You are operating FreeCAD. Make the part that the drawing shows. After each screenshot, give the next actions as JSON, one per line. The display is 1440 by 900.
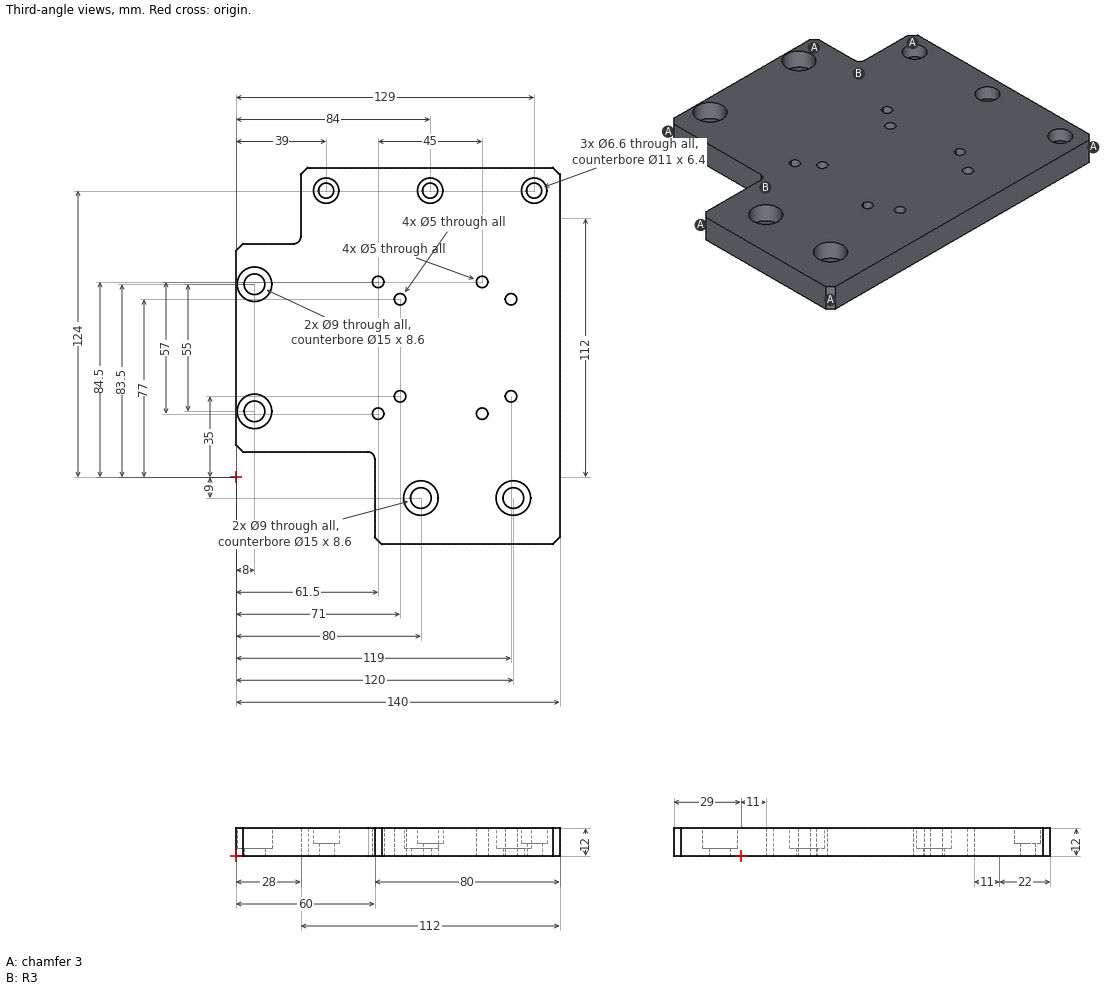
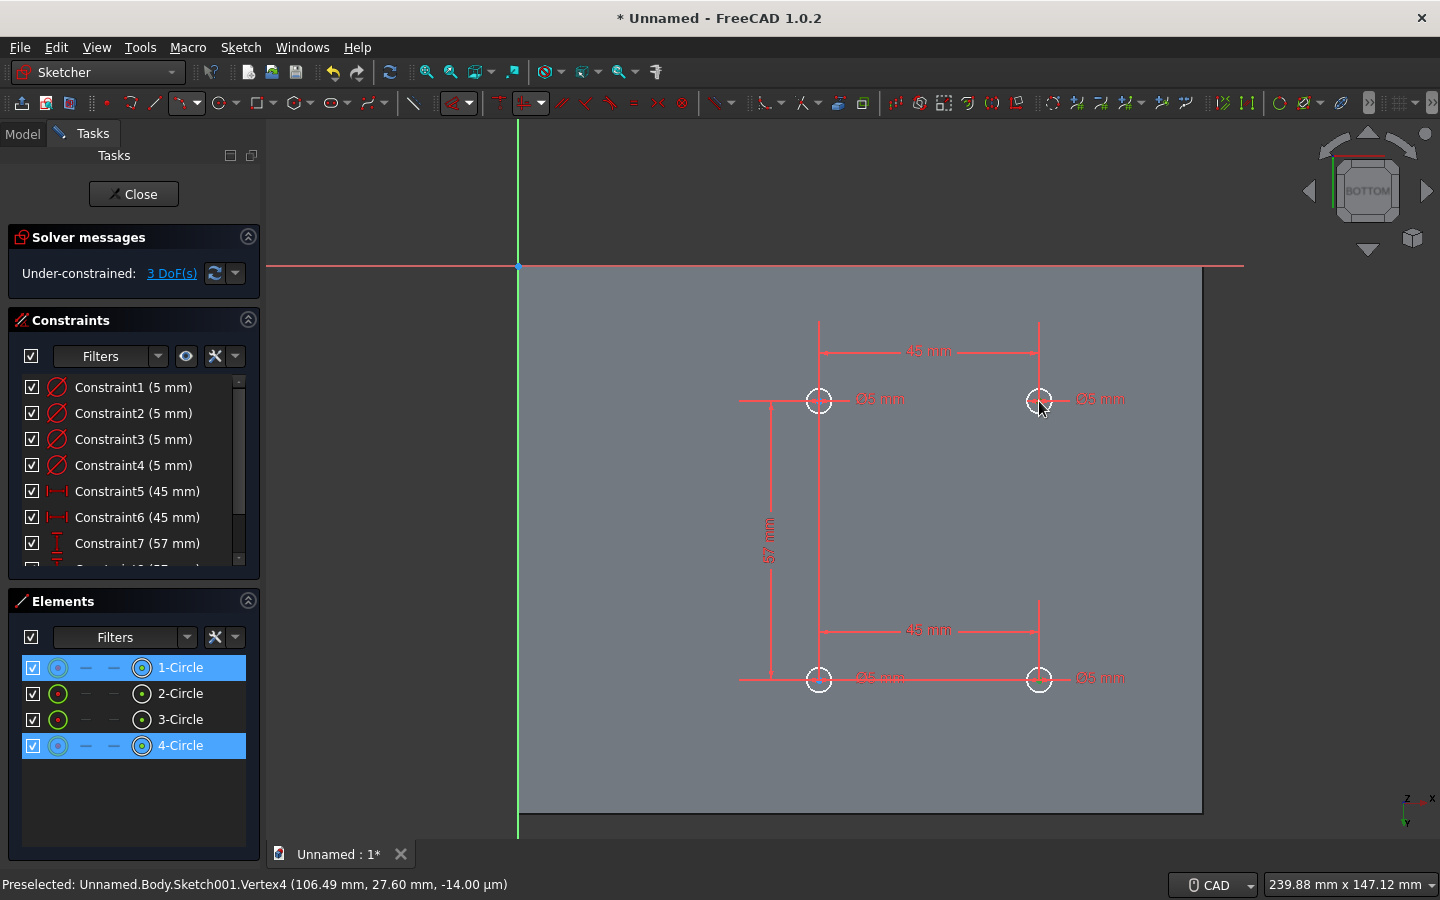
{"action": "left_click", "coordinate": [472, 104]}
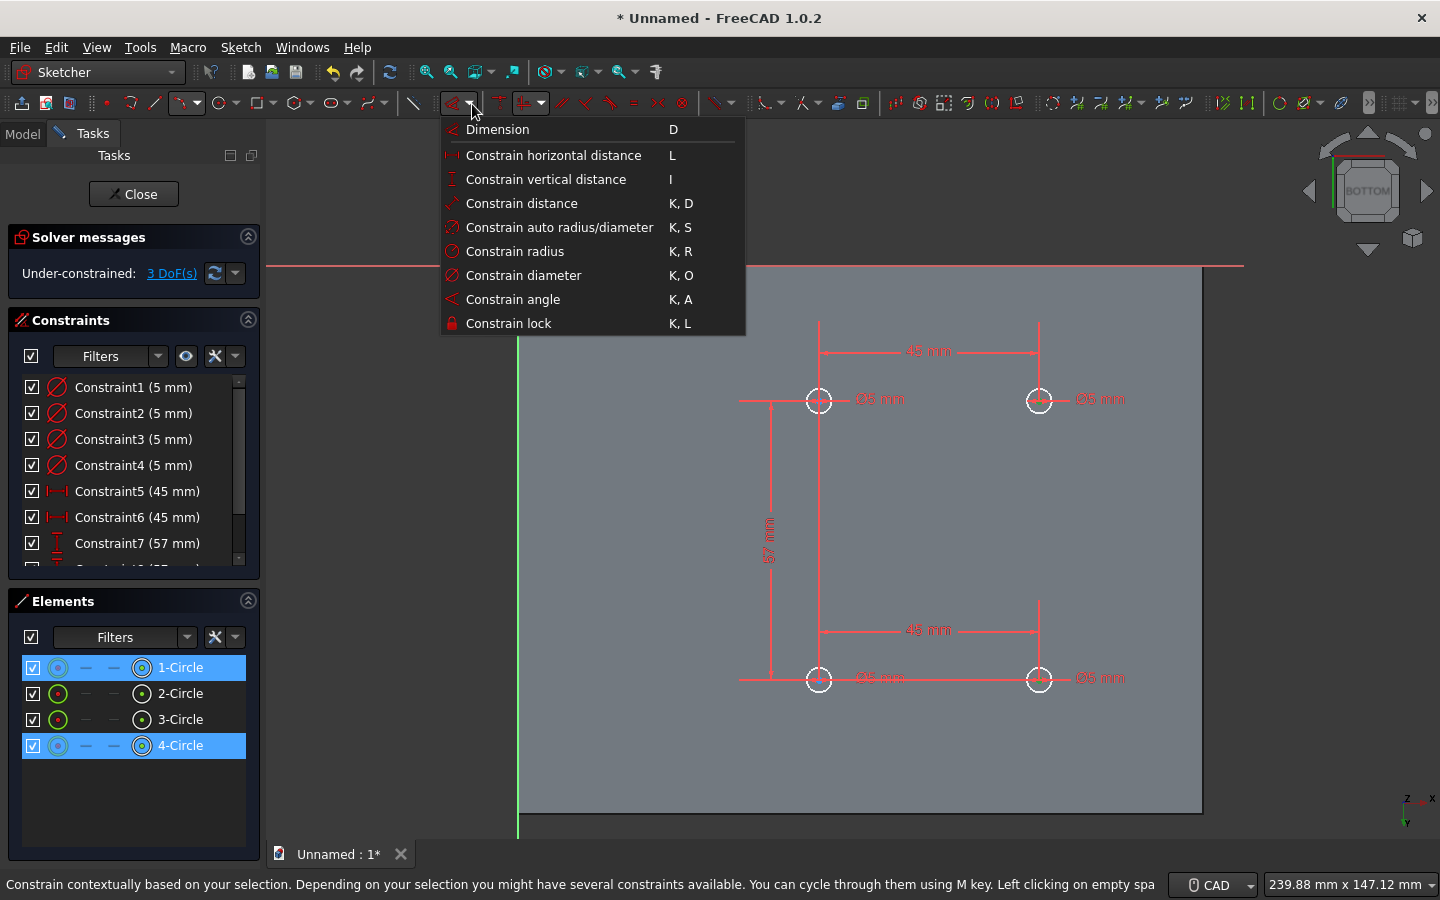
{"action": "left_click", "coordinate": [593, 179]}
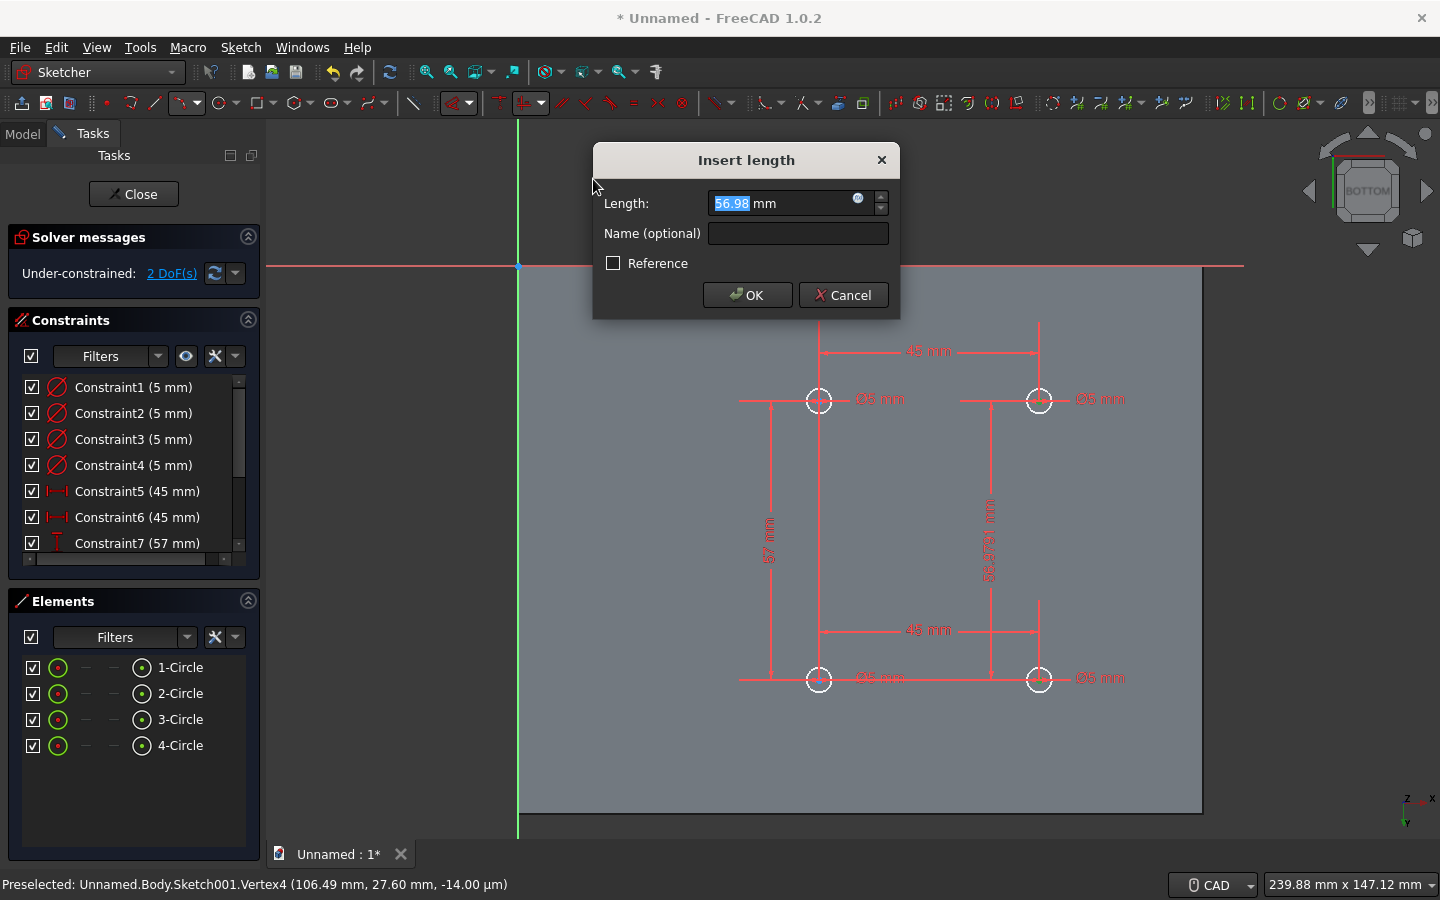
{"action": "type", "text": "57"}
{"action": "key", "text": "Return"}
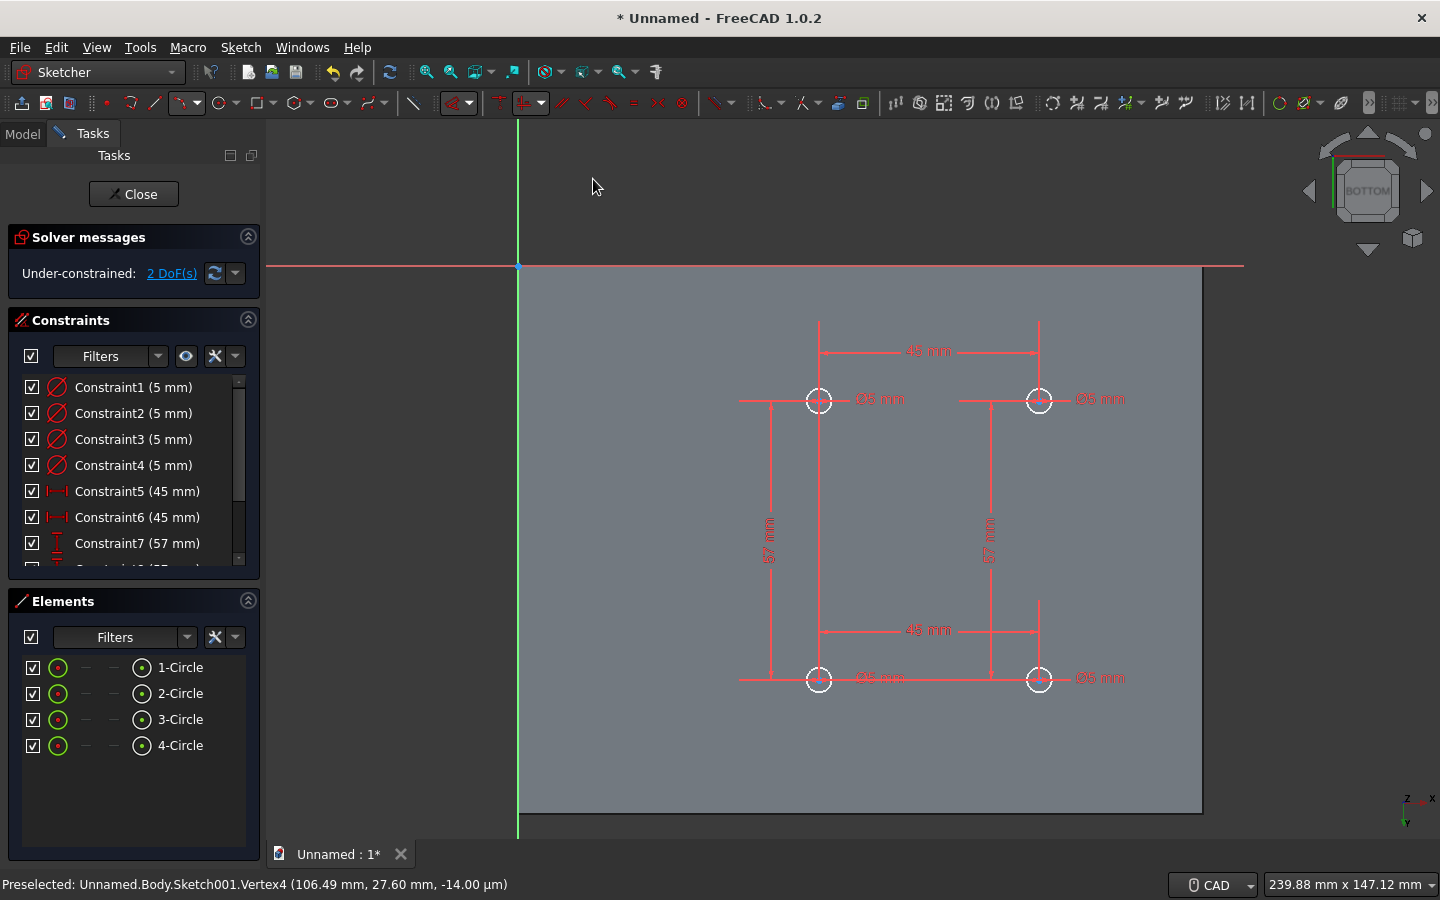
{"action": "left_click", "coordinate": [1039, 680]}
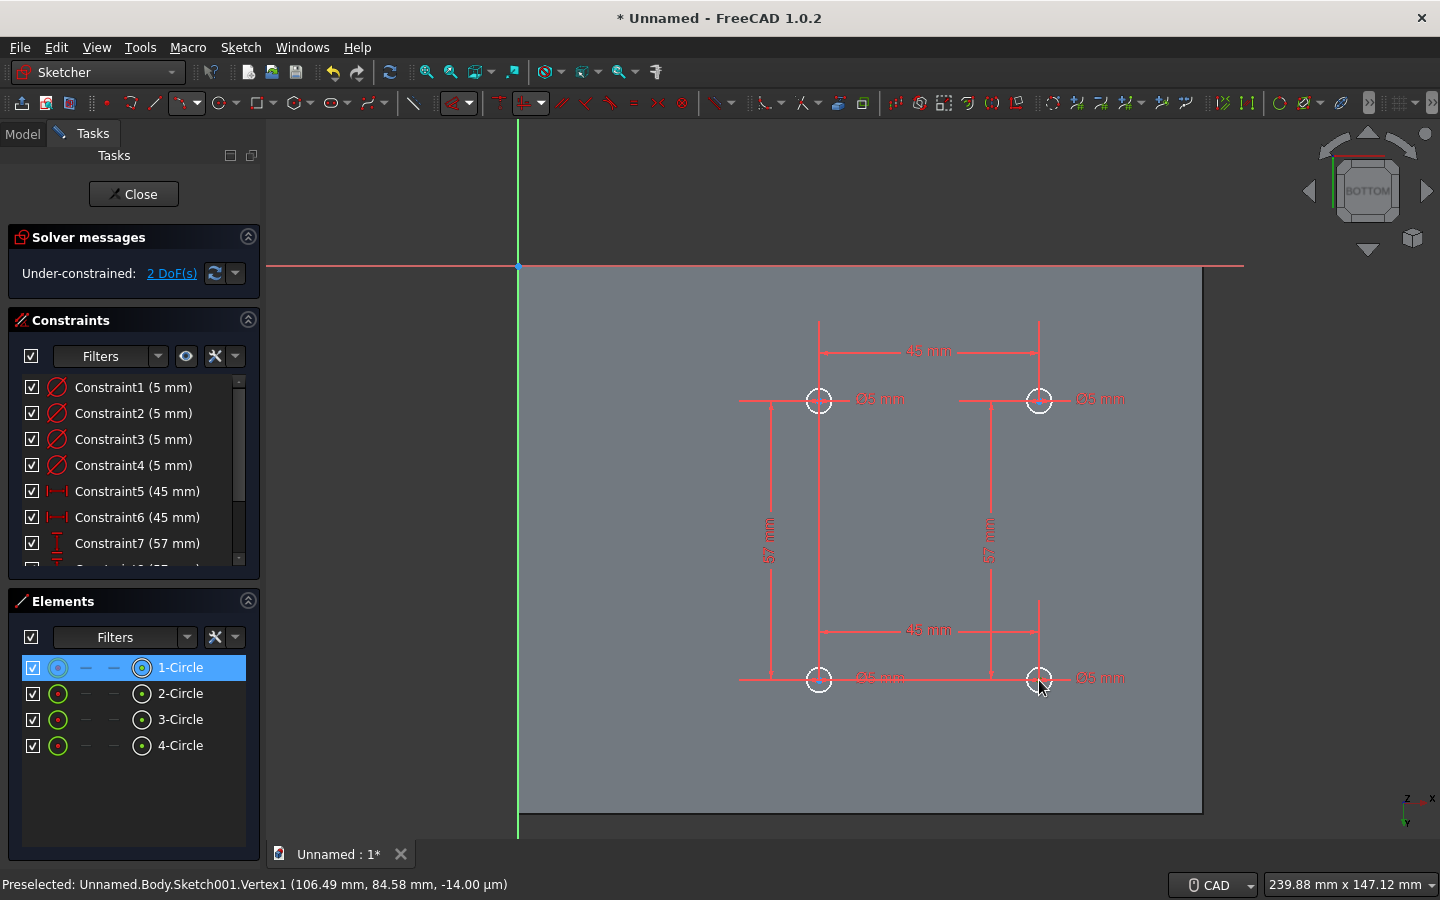
{"action": "key", "text": "i"}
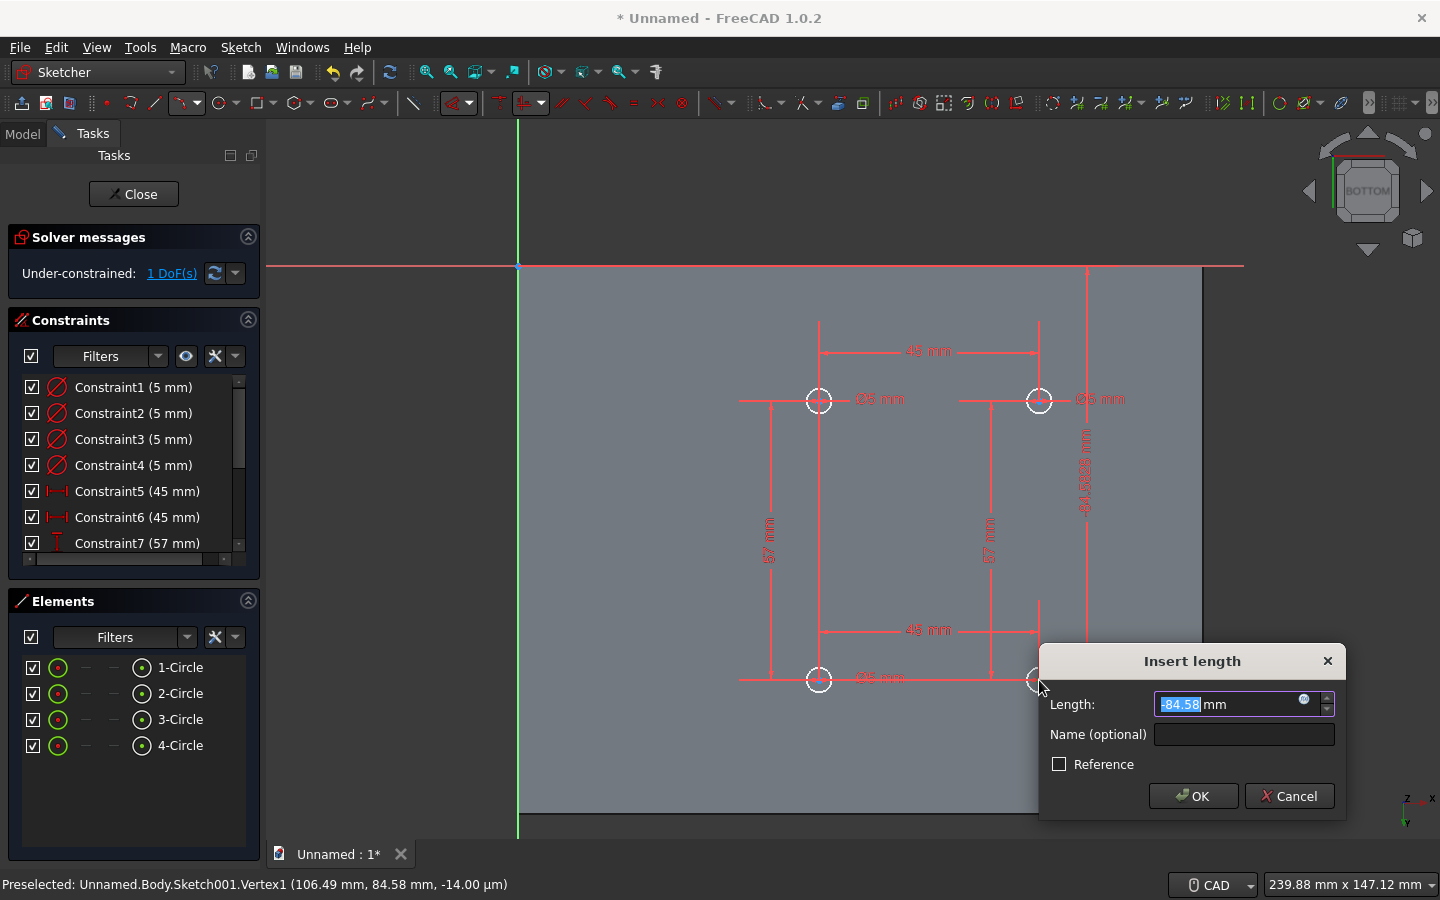
{"action": "type", "text": "-84.5"}
{"action": "key", "text": "Return"}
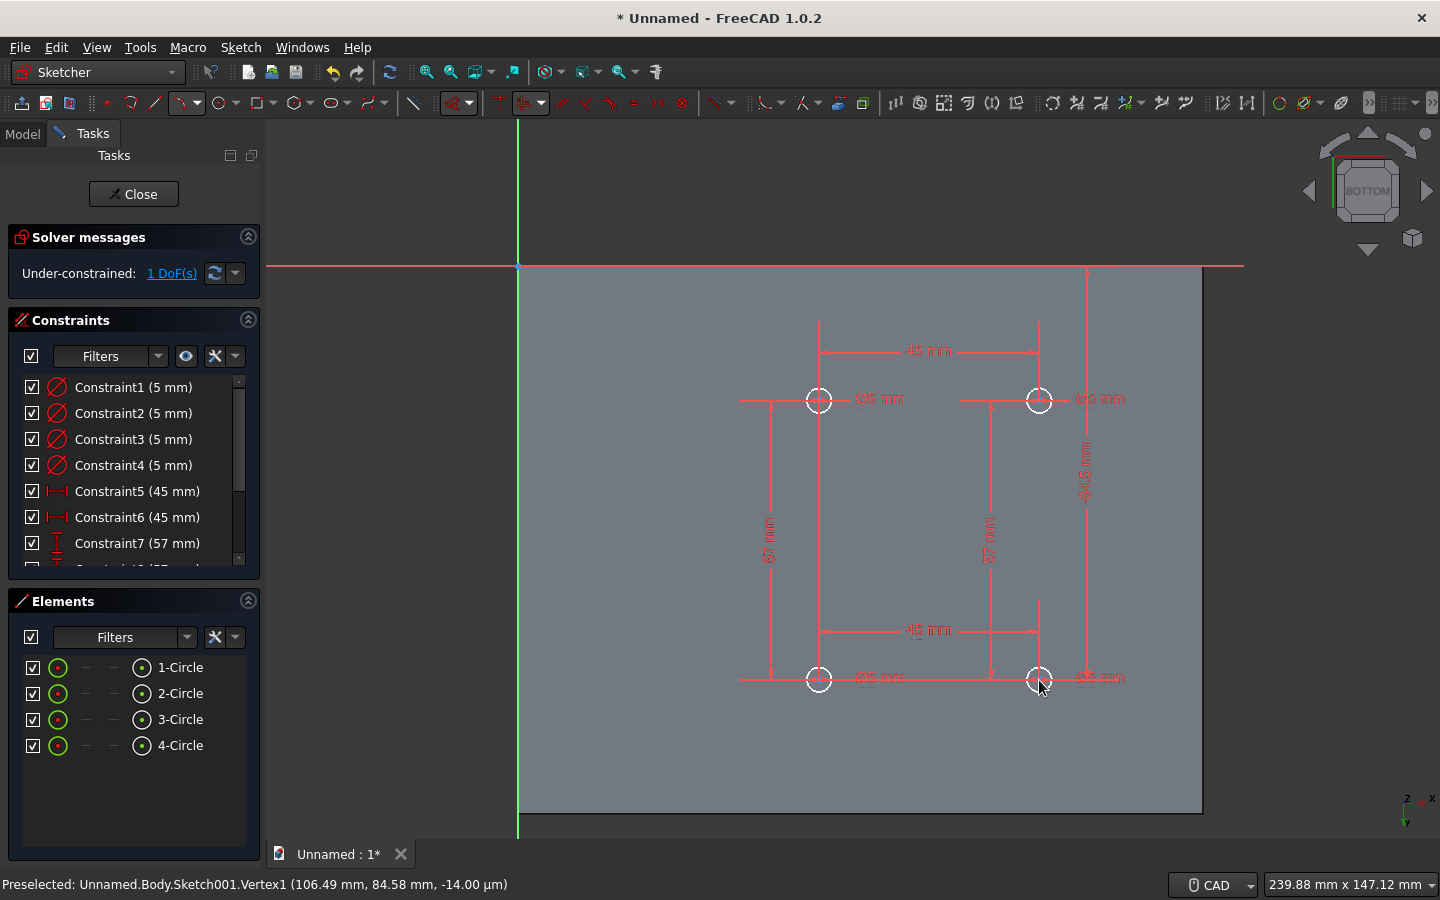
{"action": "left_click", "coordinate": [819, 680]}